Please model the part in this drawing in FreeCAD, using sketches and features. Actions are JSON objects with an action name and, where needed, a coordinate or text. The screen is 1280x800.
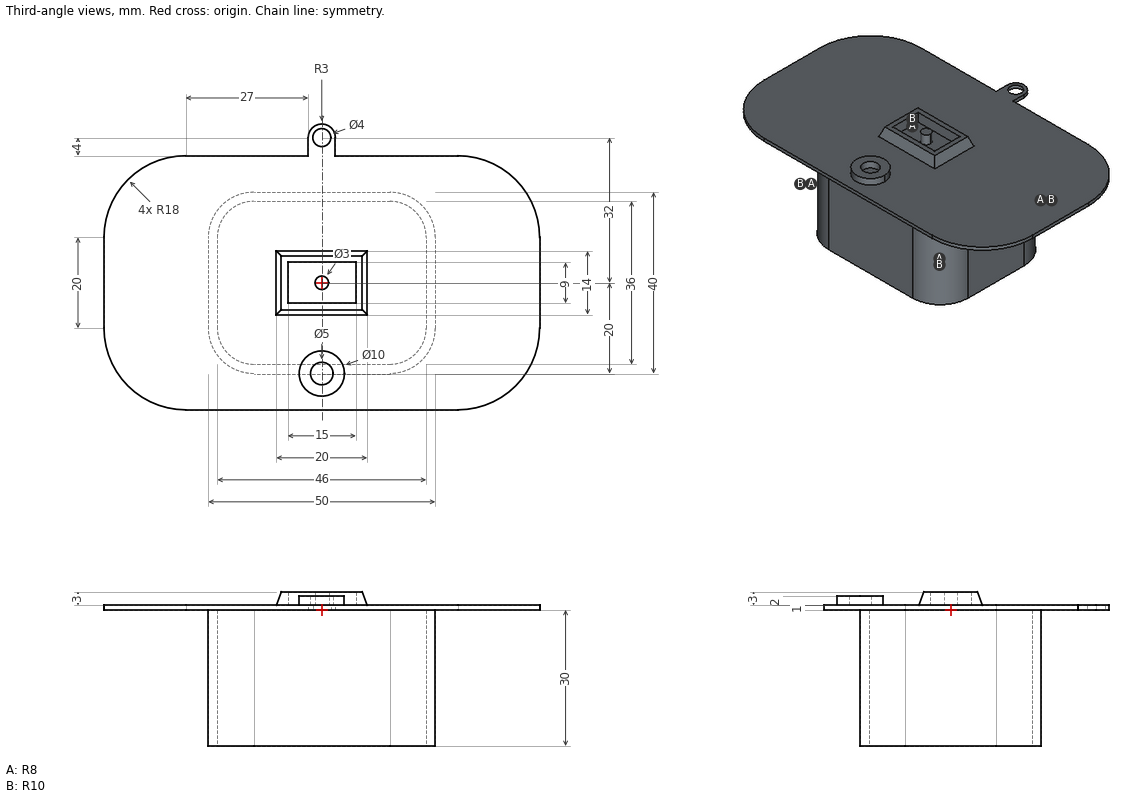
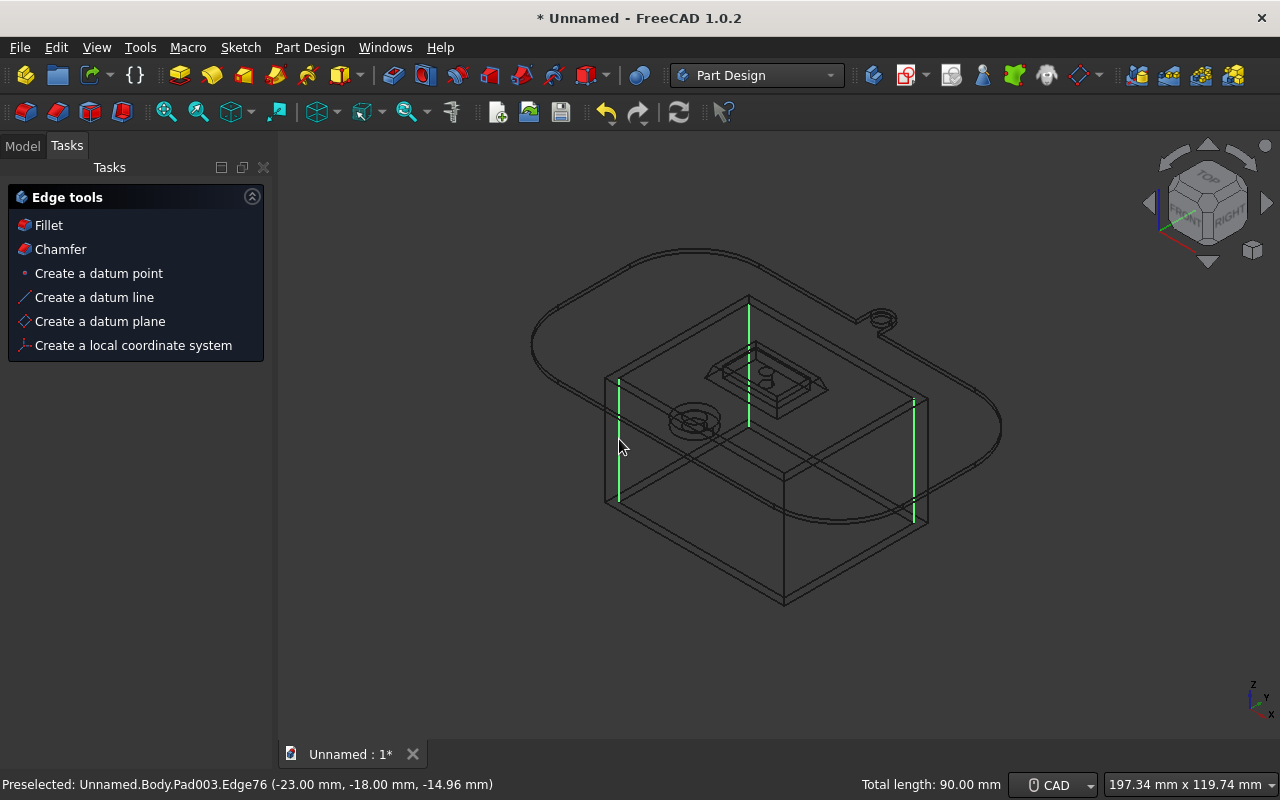
{"action": "key", "text": "2"}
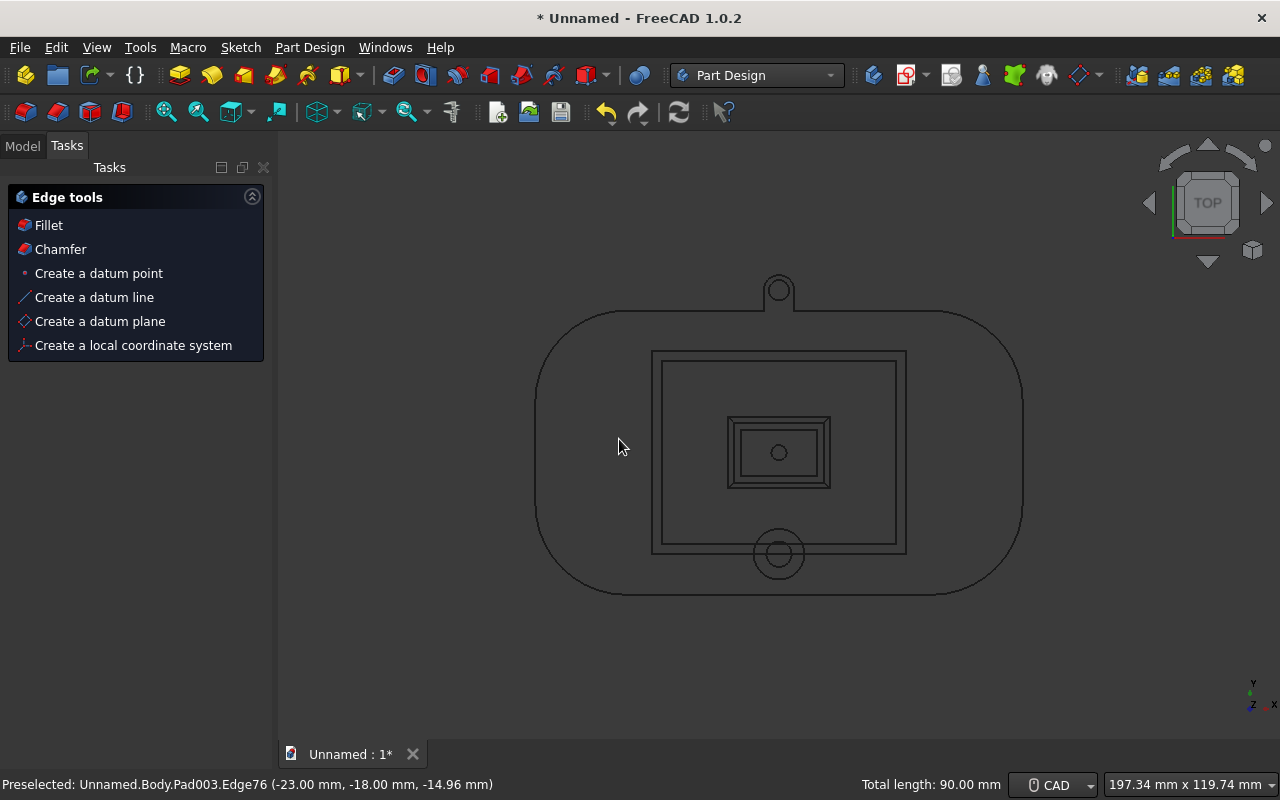
{"action": "key", "text": "1"}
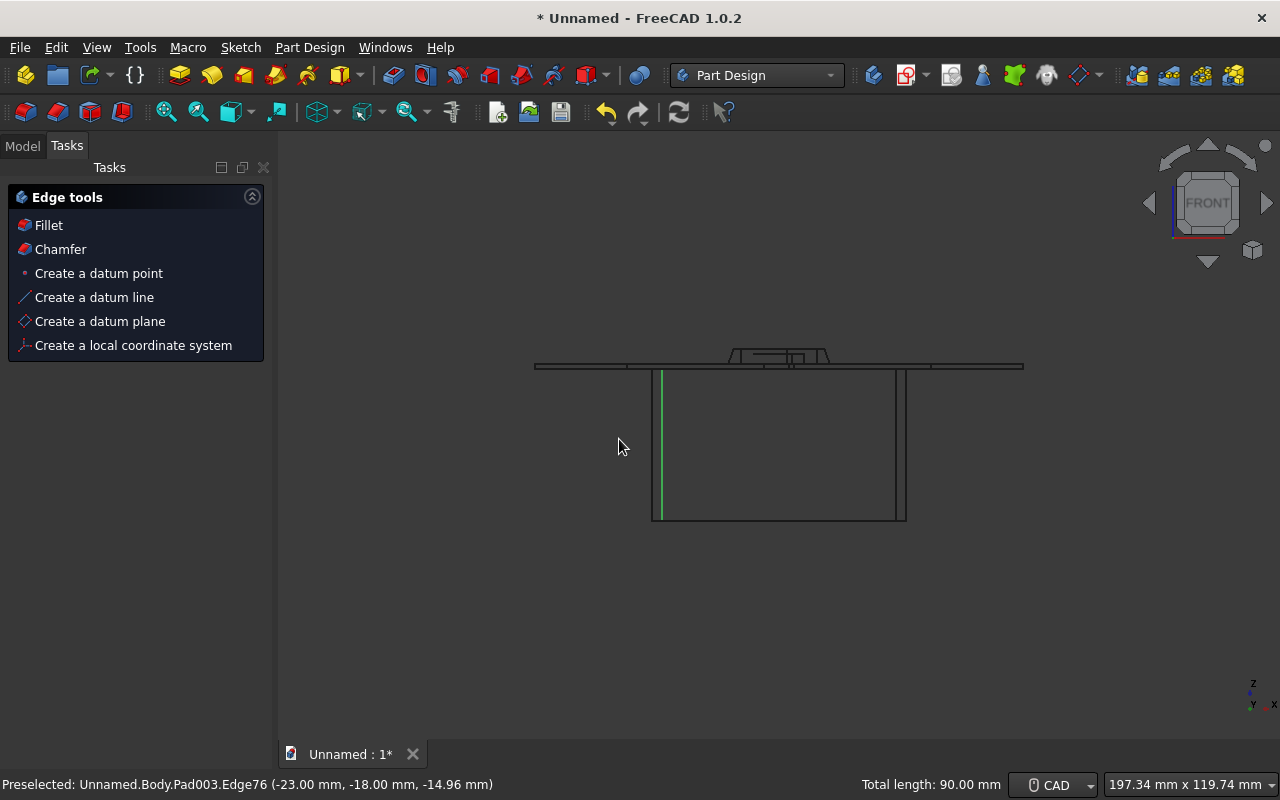
{"action": "left_click", "coordinate": [896, 444], "text": "ctrl"}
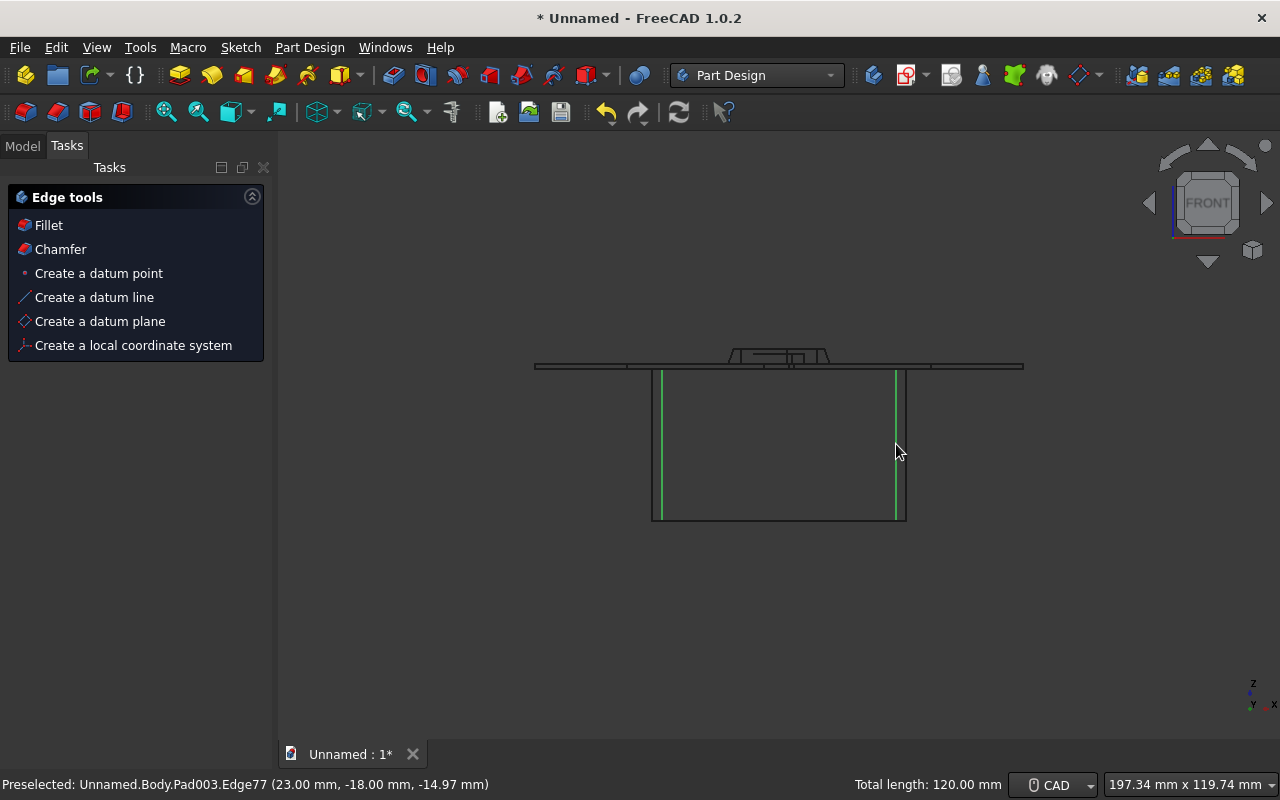
{"action": "key", "text": "v 1"}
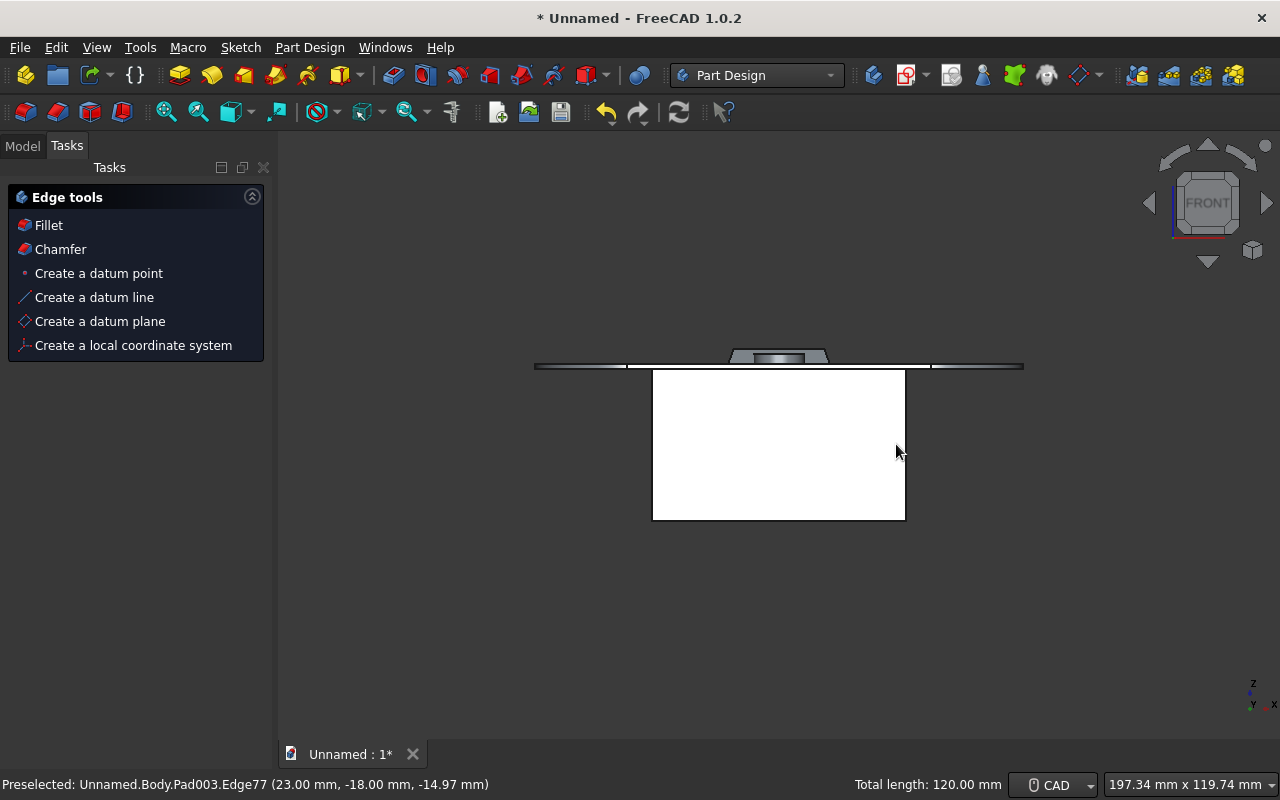
{"action": "left_click", "coordinate": [26, 112]}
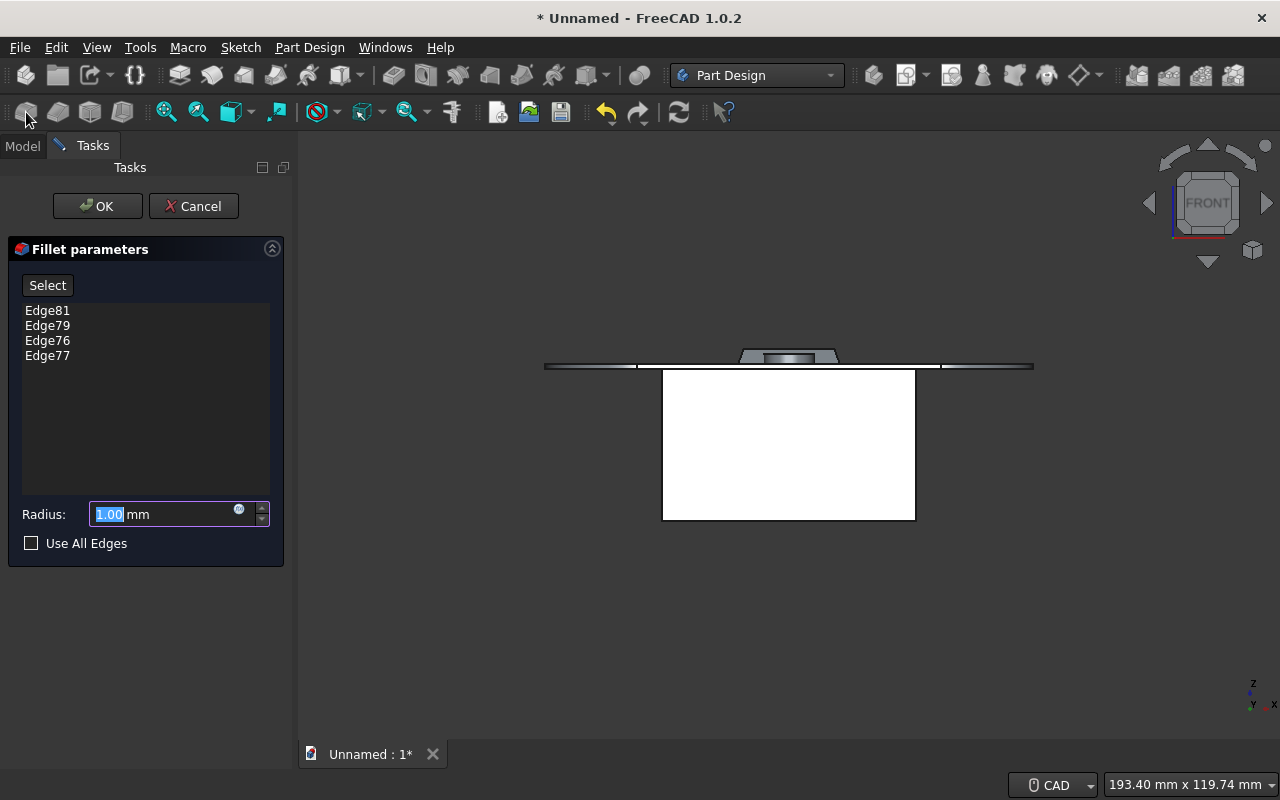
{"action": "type", "text": "8"}
{"action": "key", "text": "Tab"}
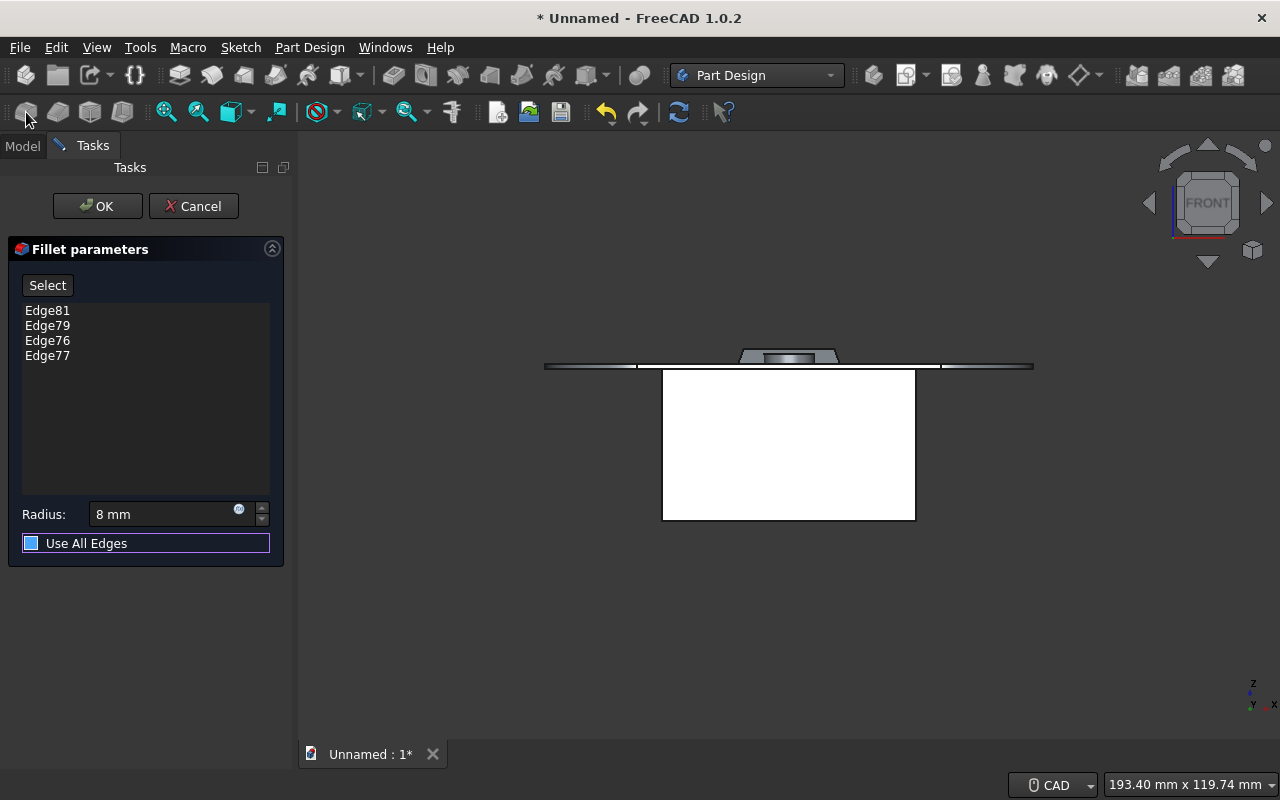
{"action": "left_click", "coordinate": [98, 206]}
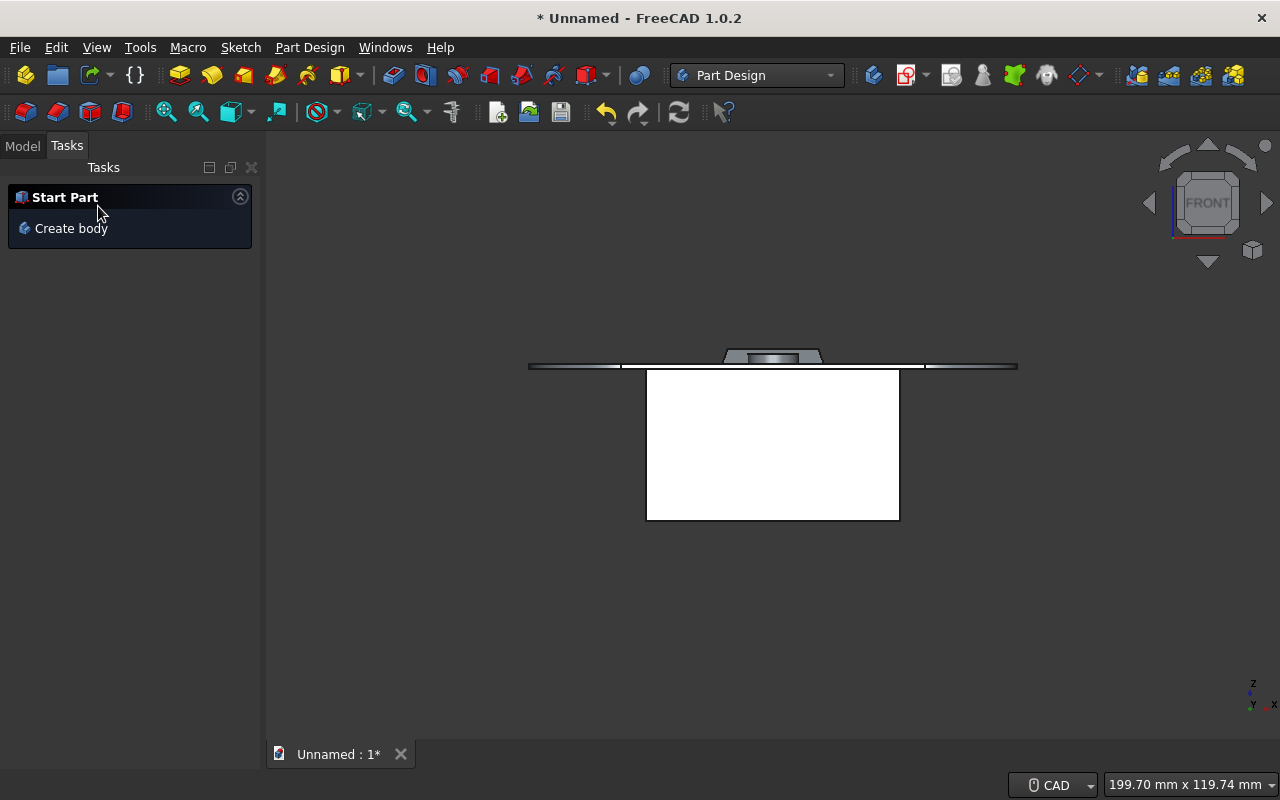
{"action": "left_click", "coordinate": [646, 444]}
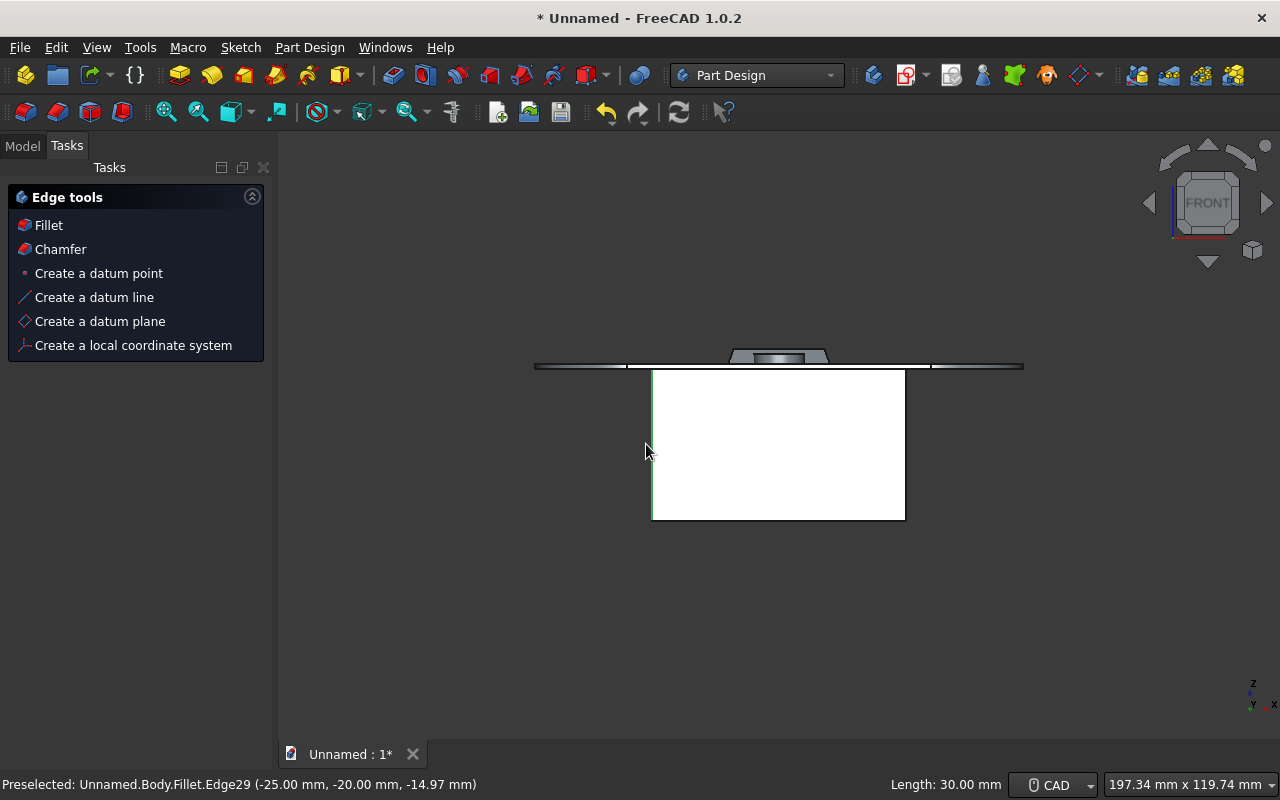
{"action": "left_click", "coordinate": [906, 444], "text": "ctrl"}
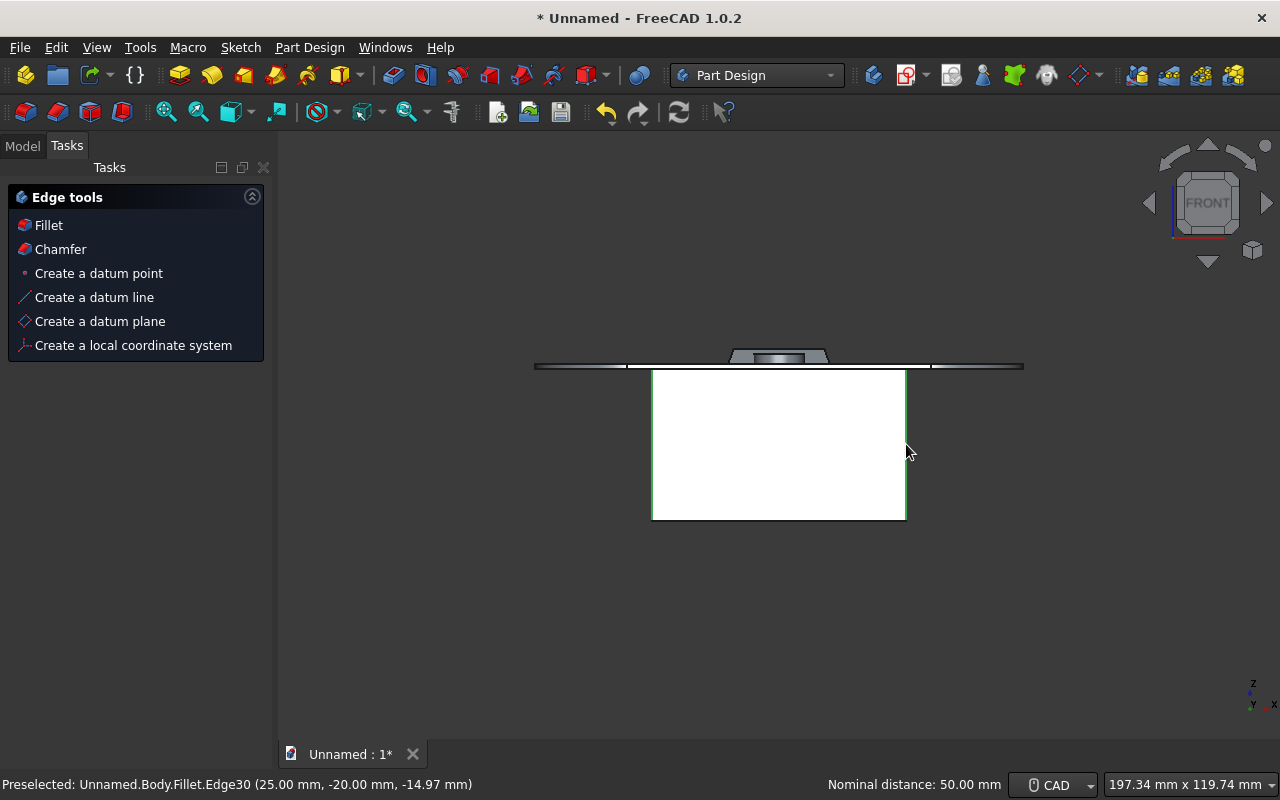
{"action": "key", "text": "0"}